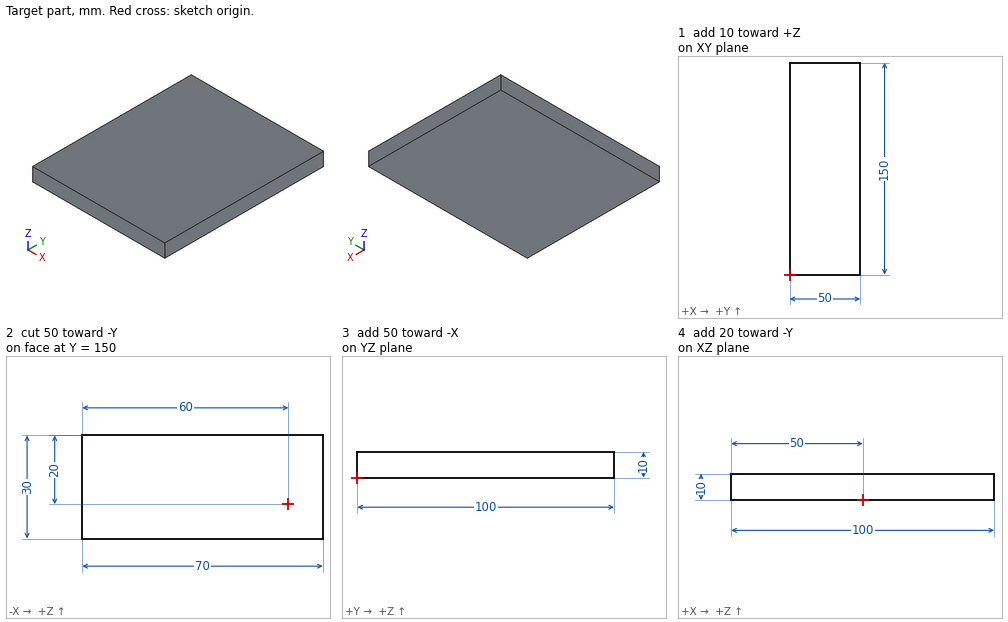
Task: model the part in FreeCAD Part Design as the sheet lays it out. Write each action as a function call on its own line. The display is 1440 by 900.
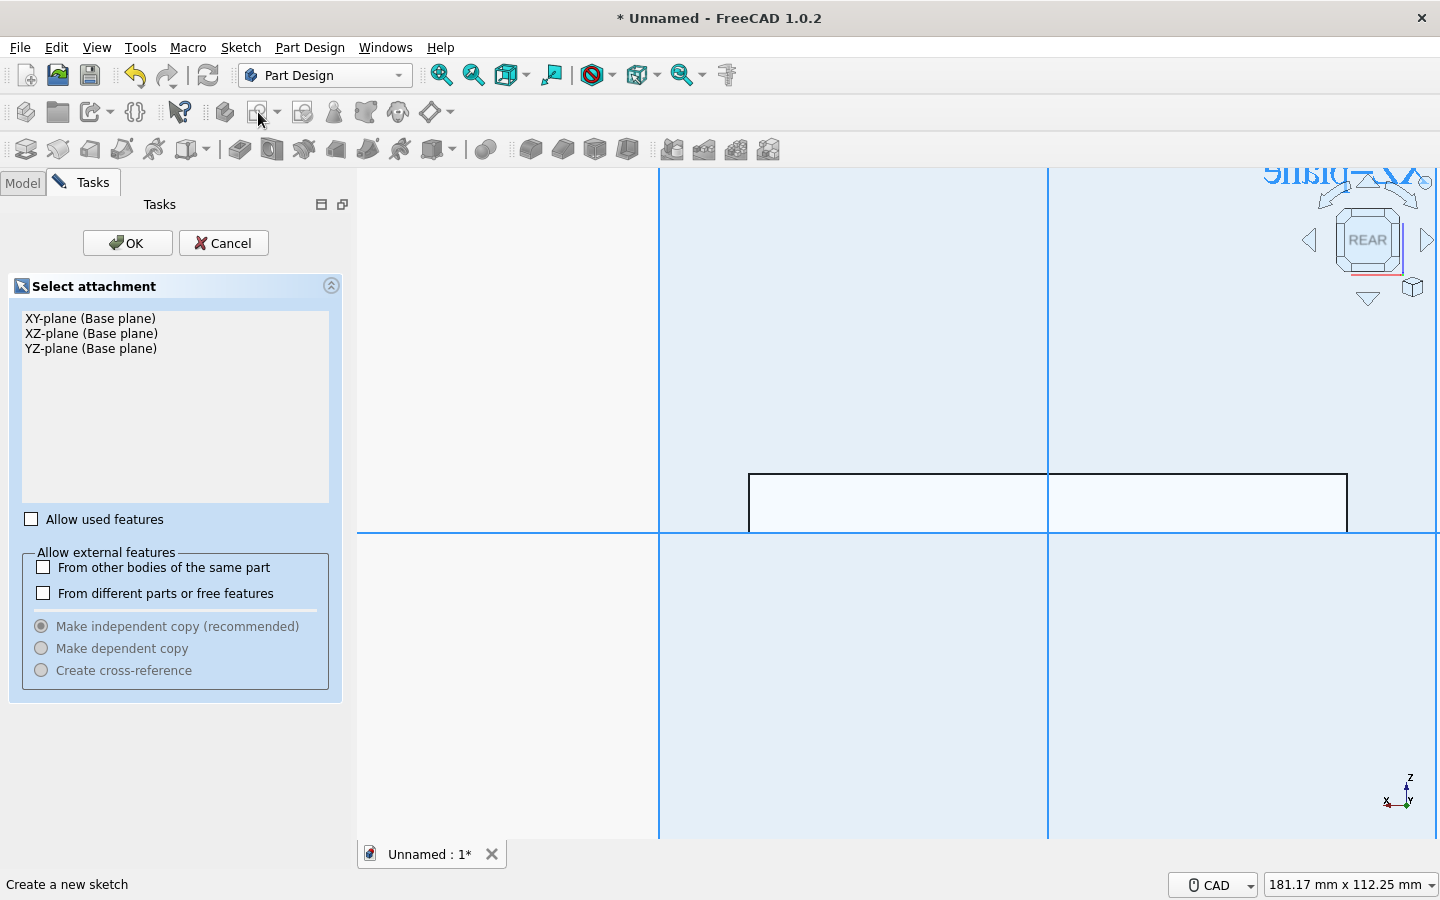
click(82, 334)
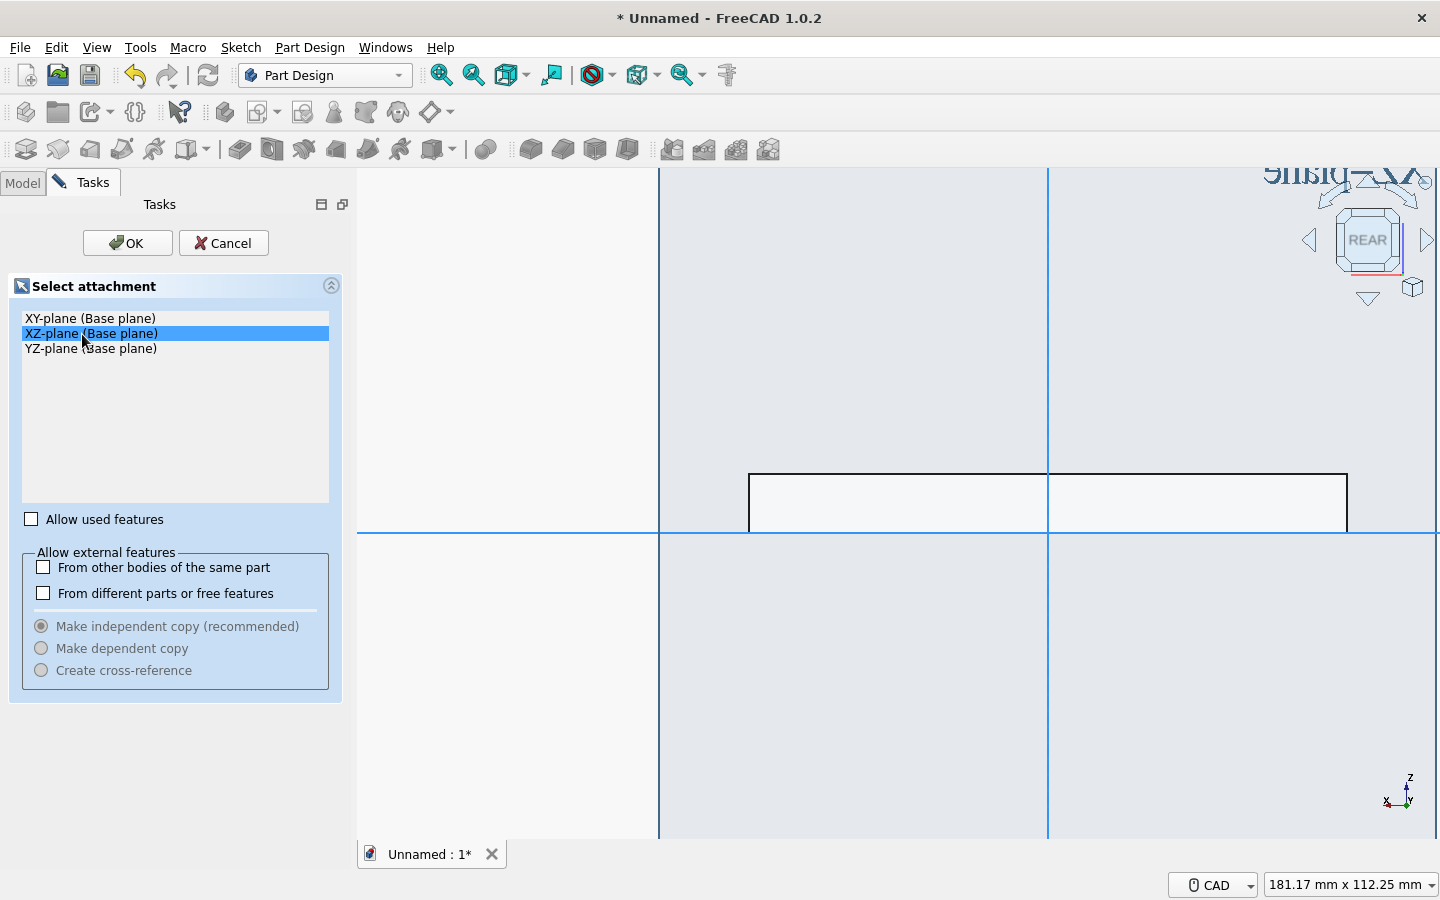
click(128, 243)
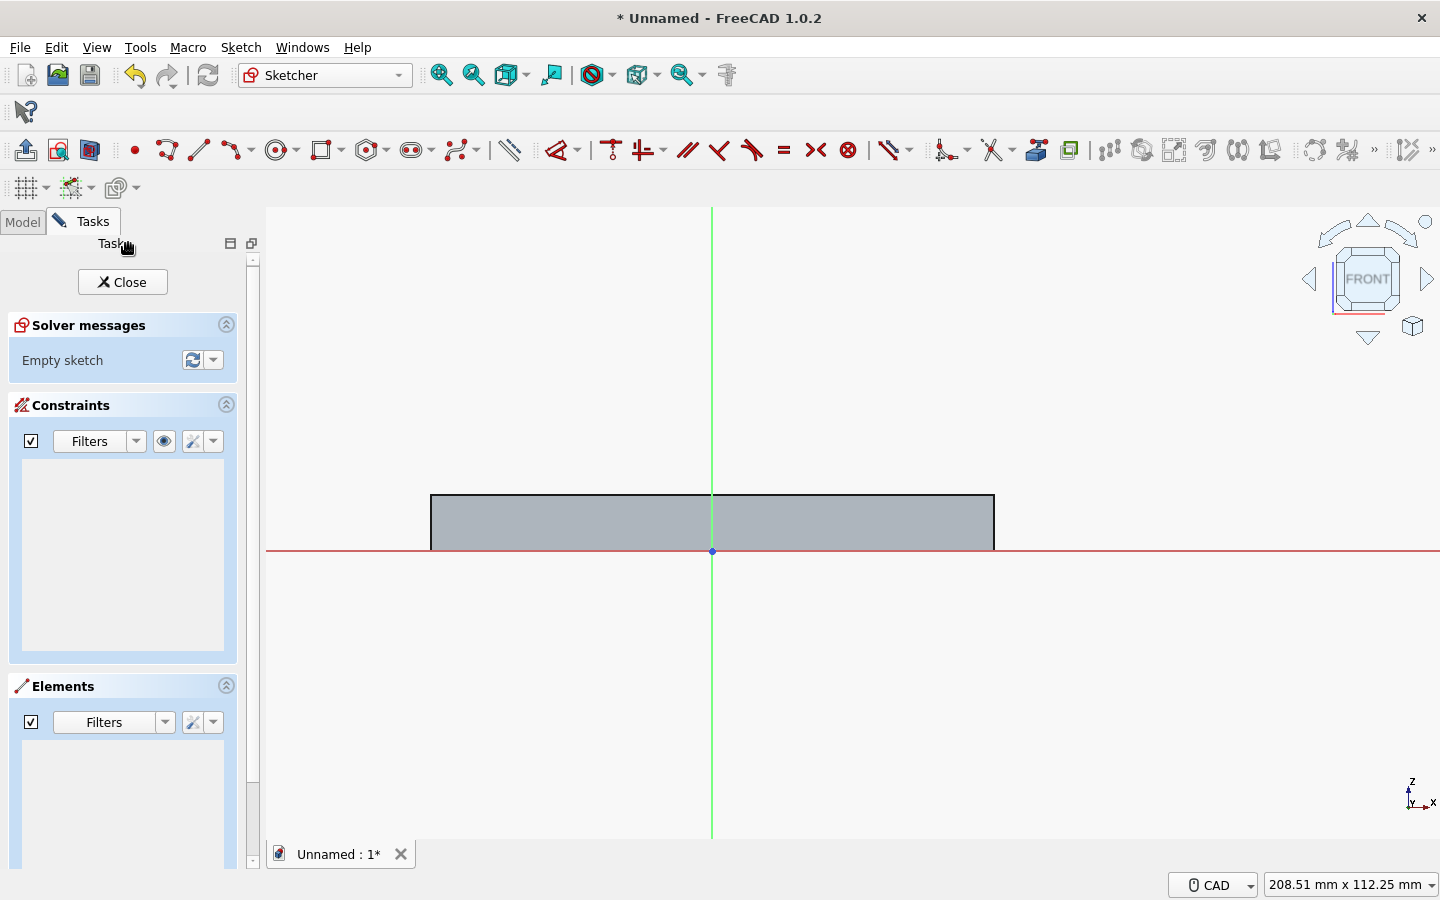
click(322, 150)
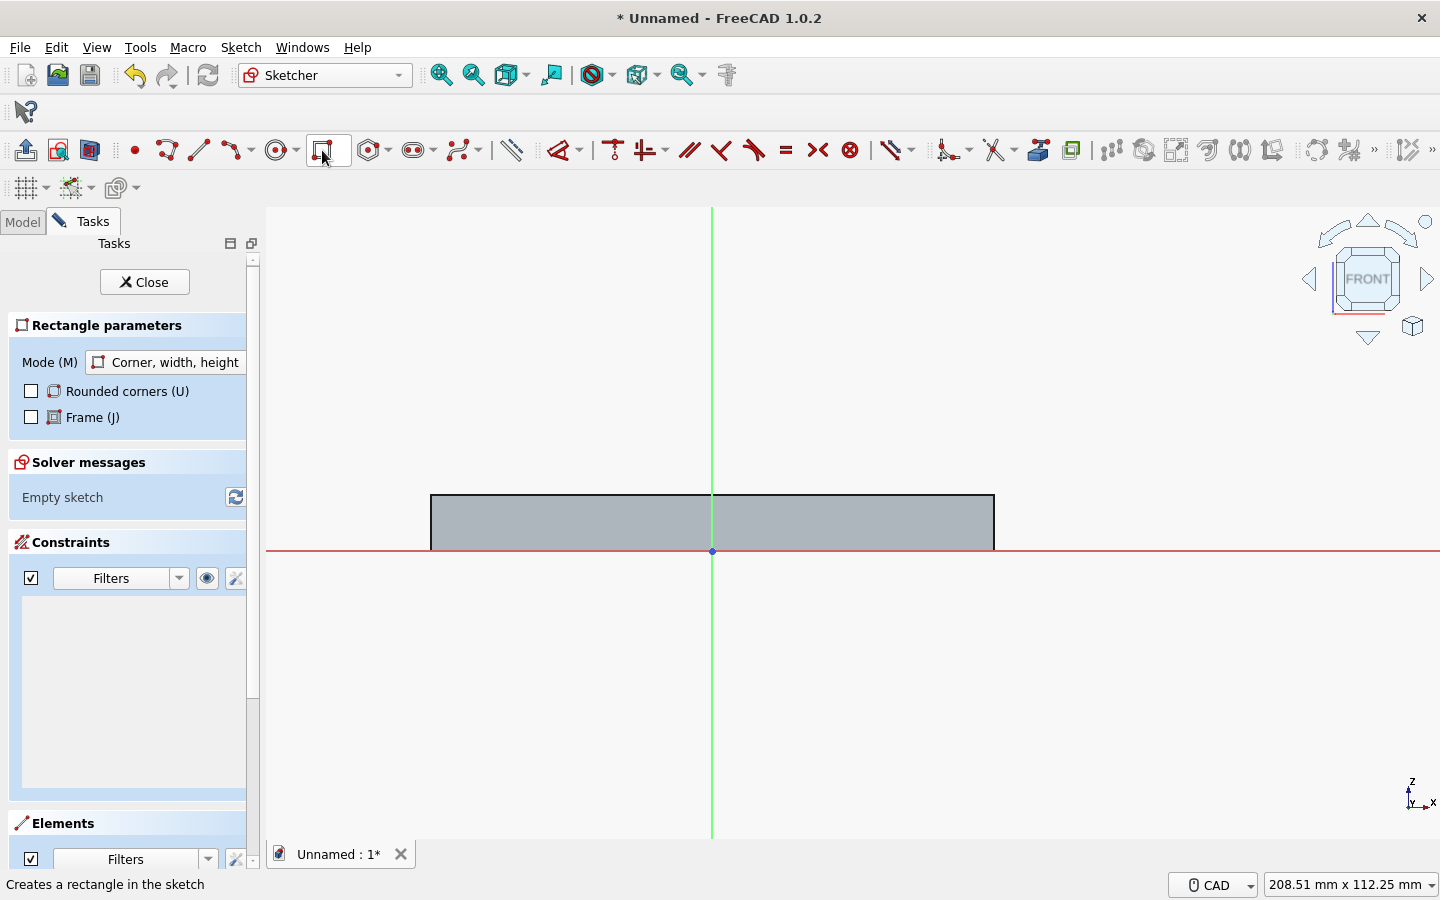
click(431, 495)
click(994, 551)
key(Escape)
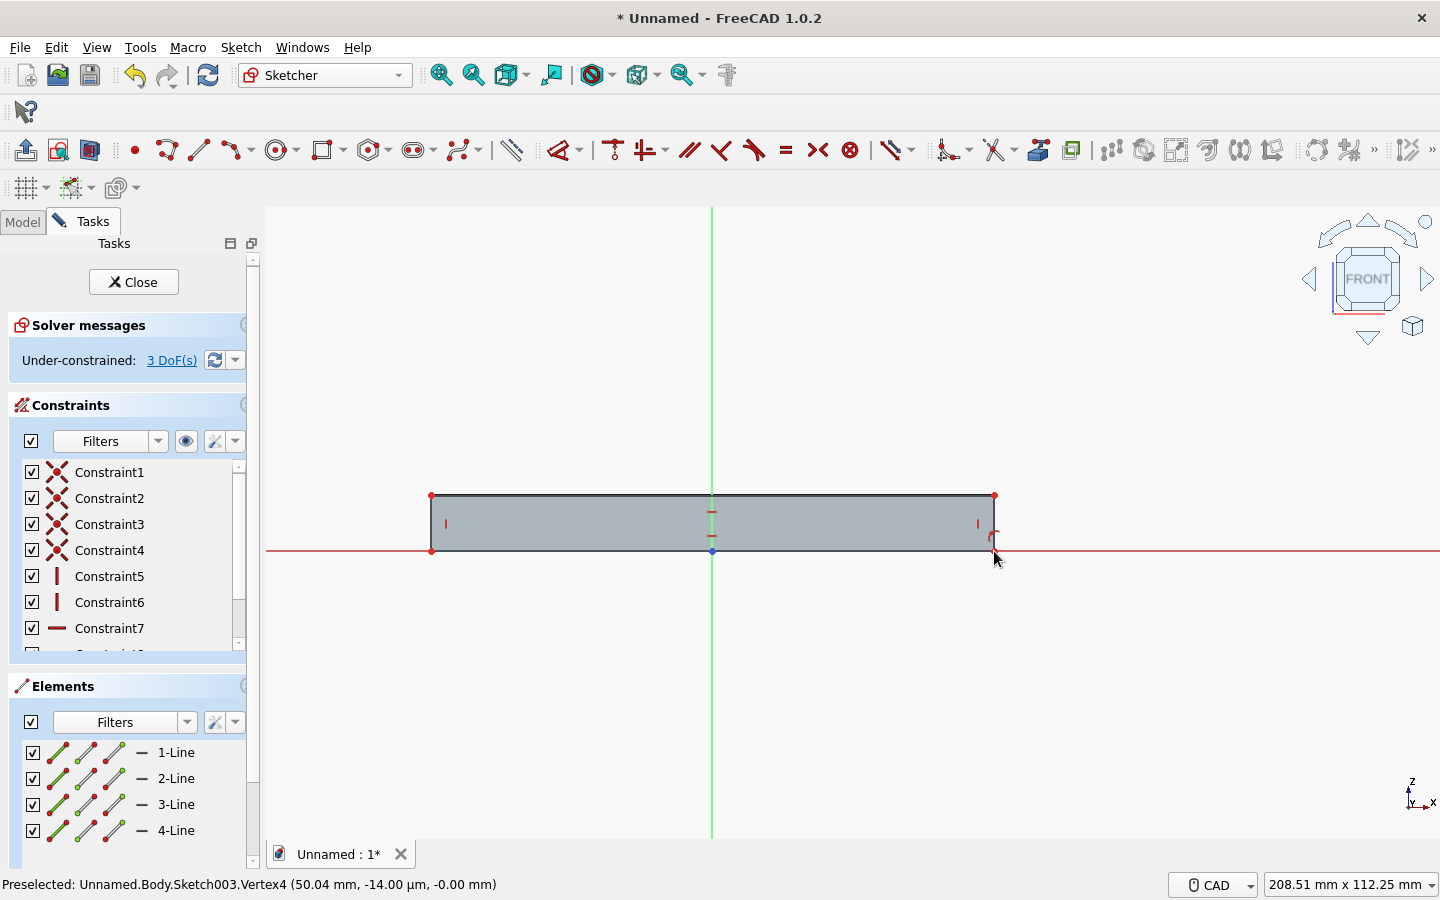
click(558, 150)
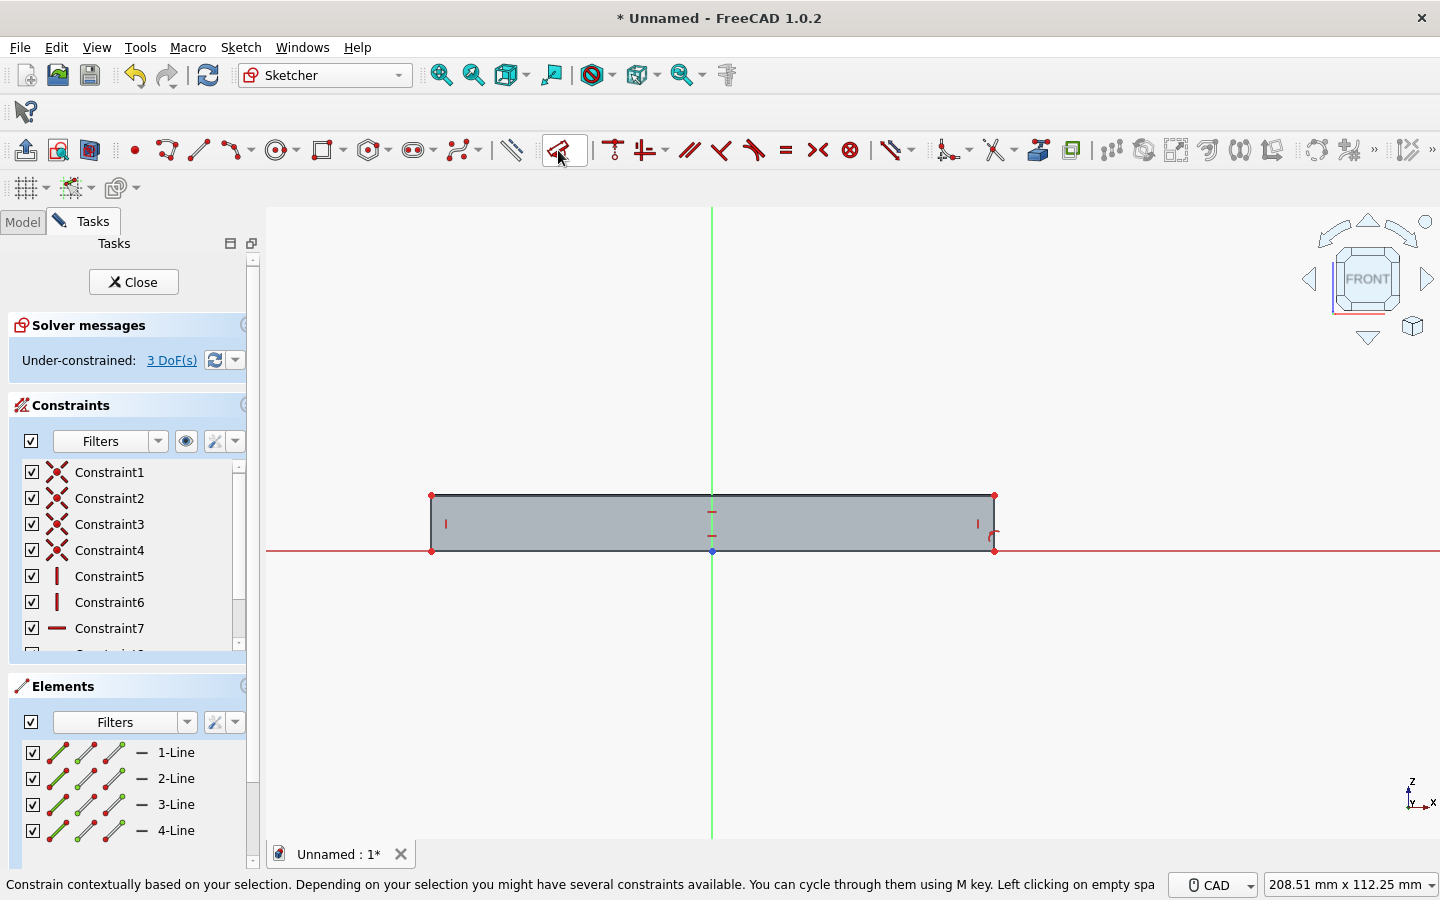
click(431, 513)
click(397, 524)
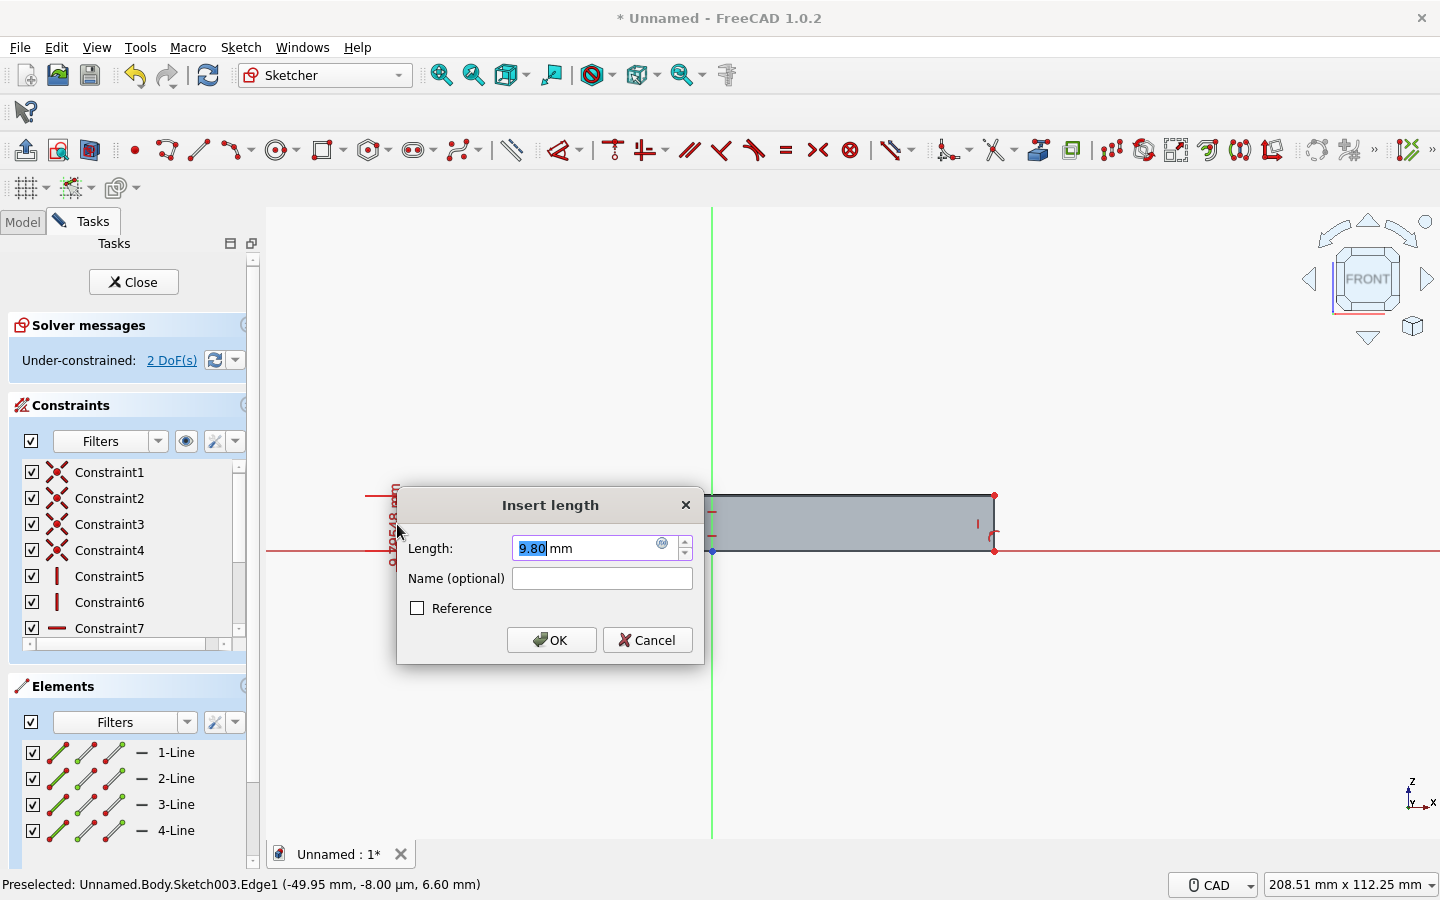
text(10)
key(Return)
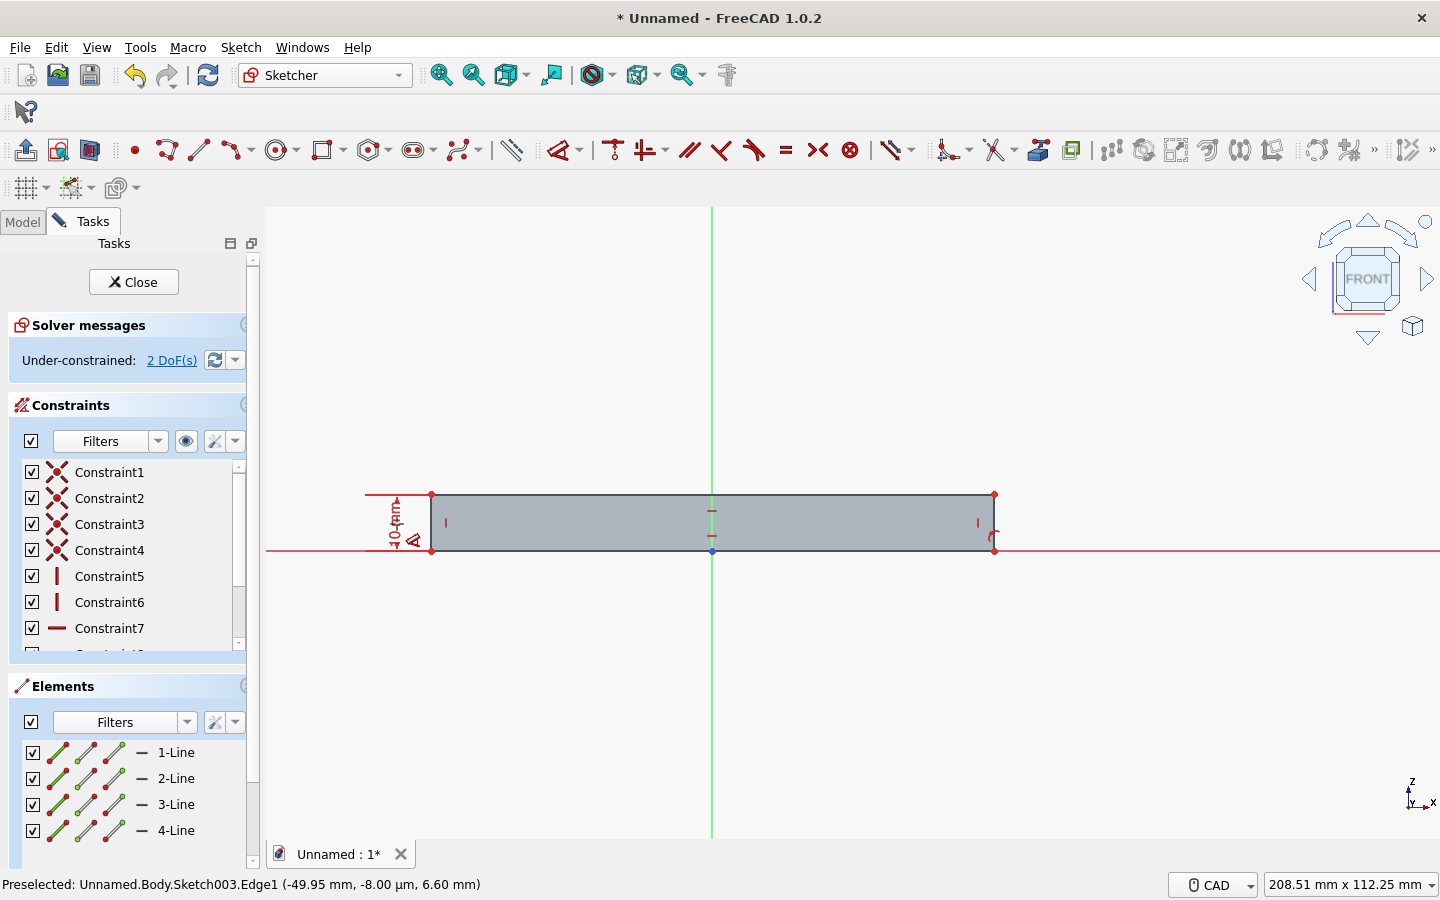
click(600, 551)
click(583, 585)